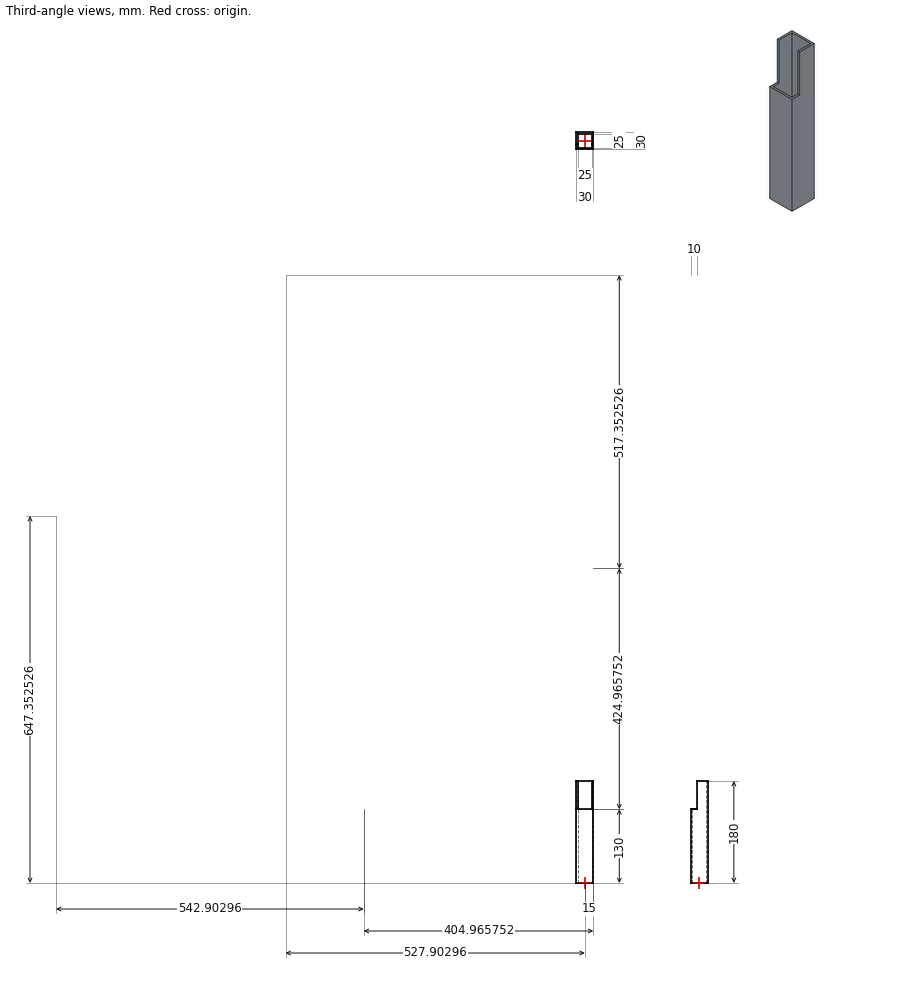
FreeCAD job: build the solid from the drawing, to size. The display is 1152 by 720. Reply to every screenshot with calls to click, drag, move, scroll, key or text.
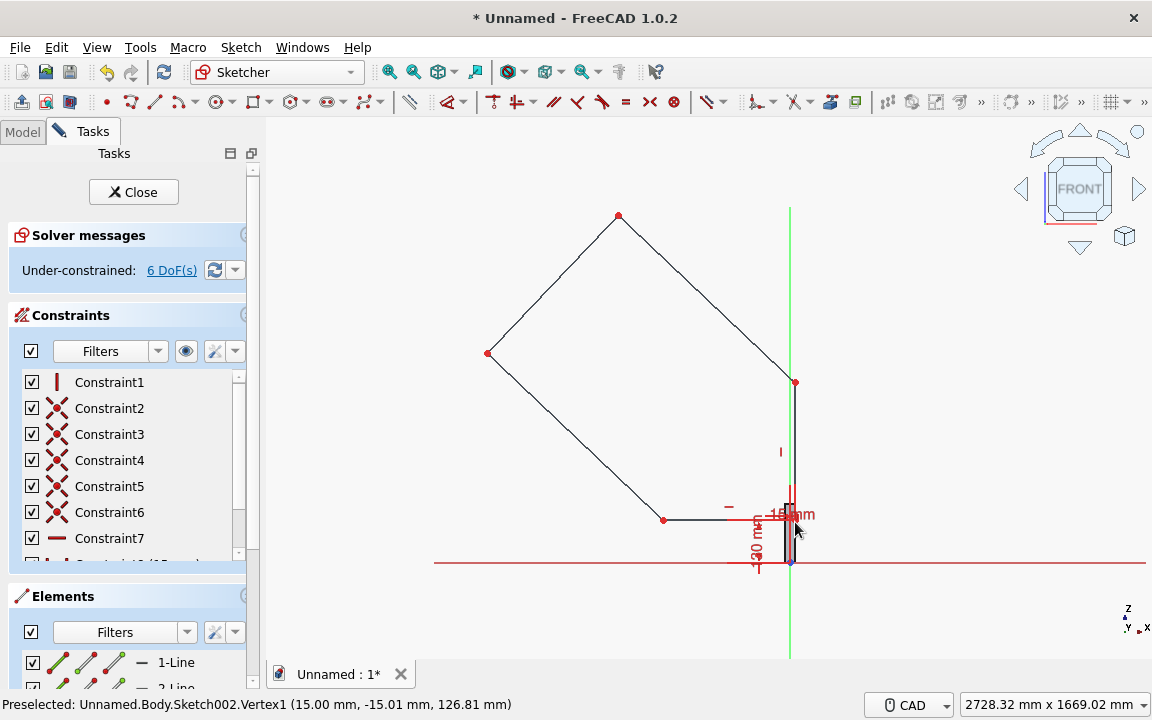
scroll(795, 479, up, 6)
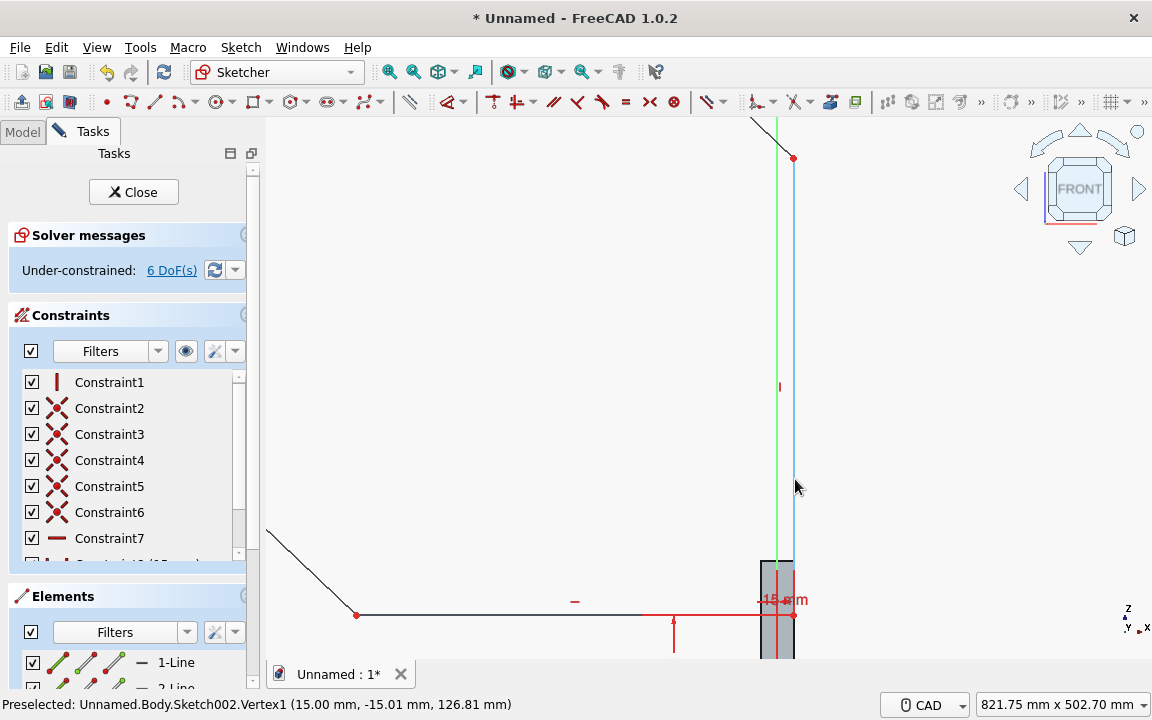
click(794, 478)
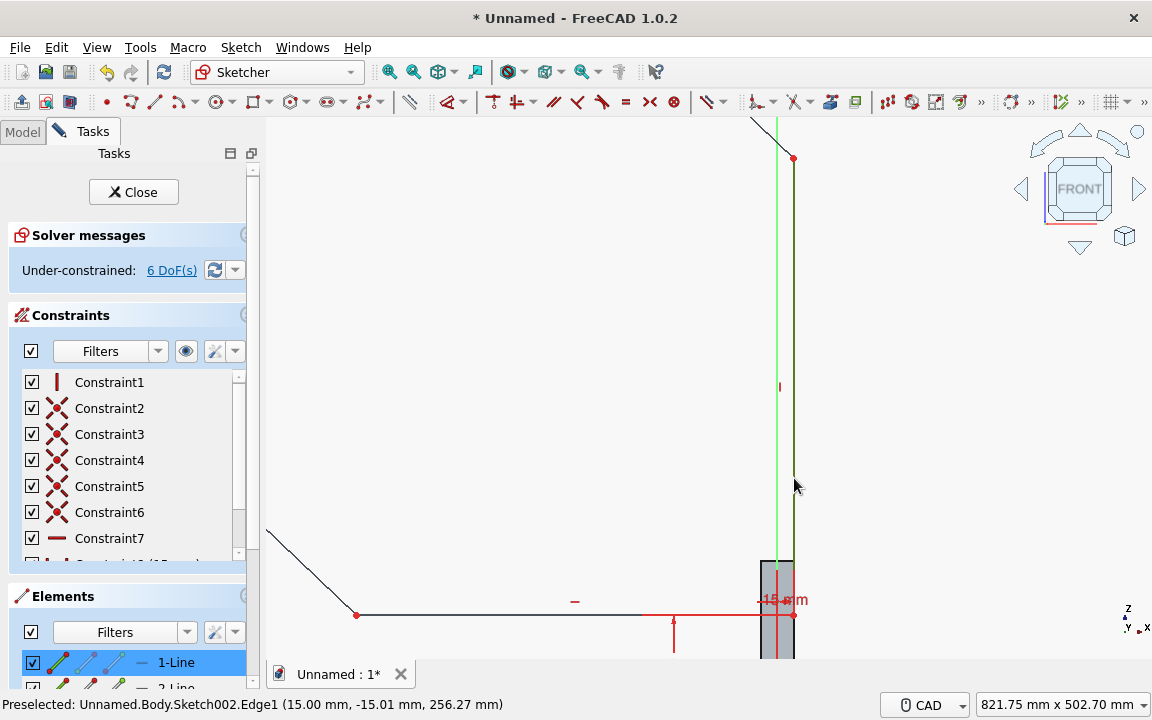
click(466, 102)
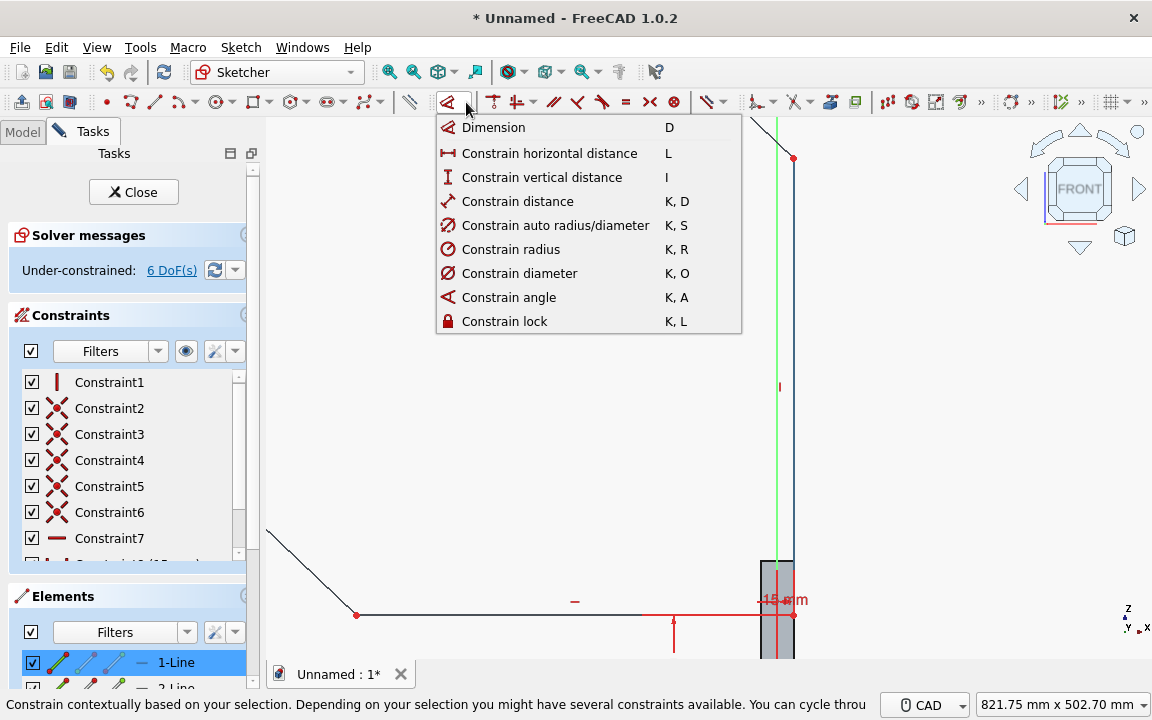
click(589, 177)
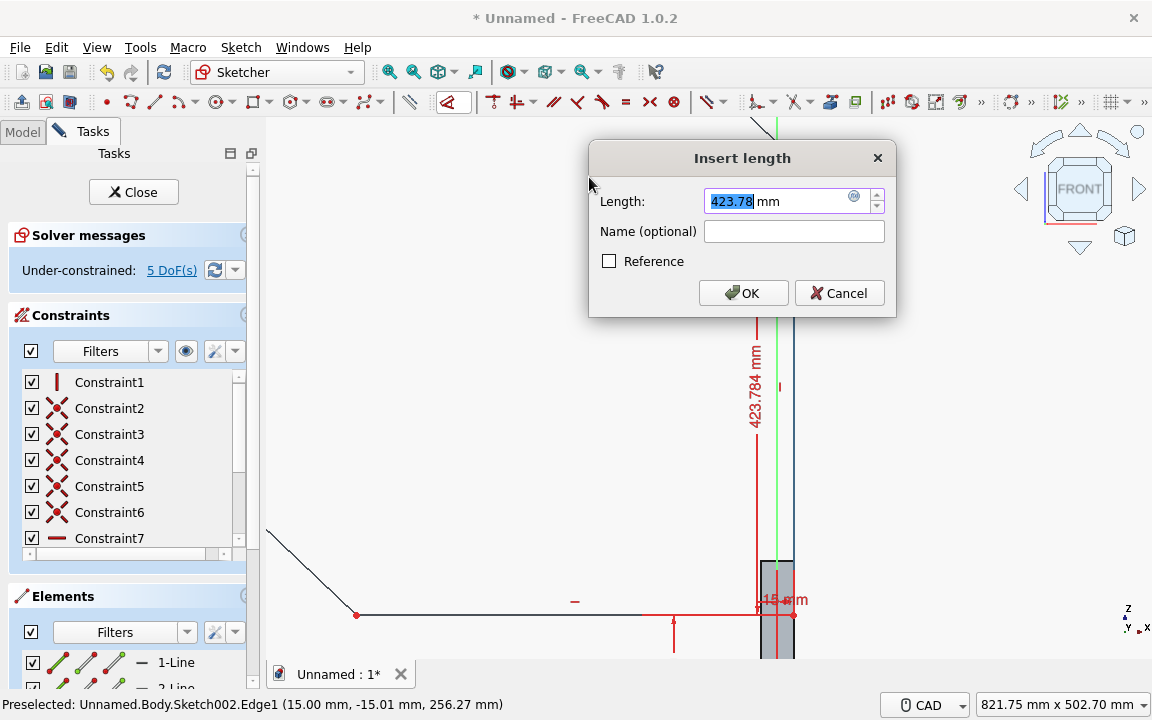
text(424.965752)
key(Return)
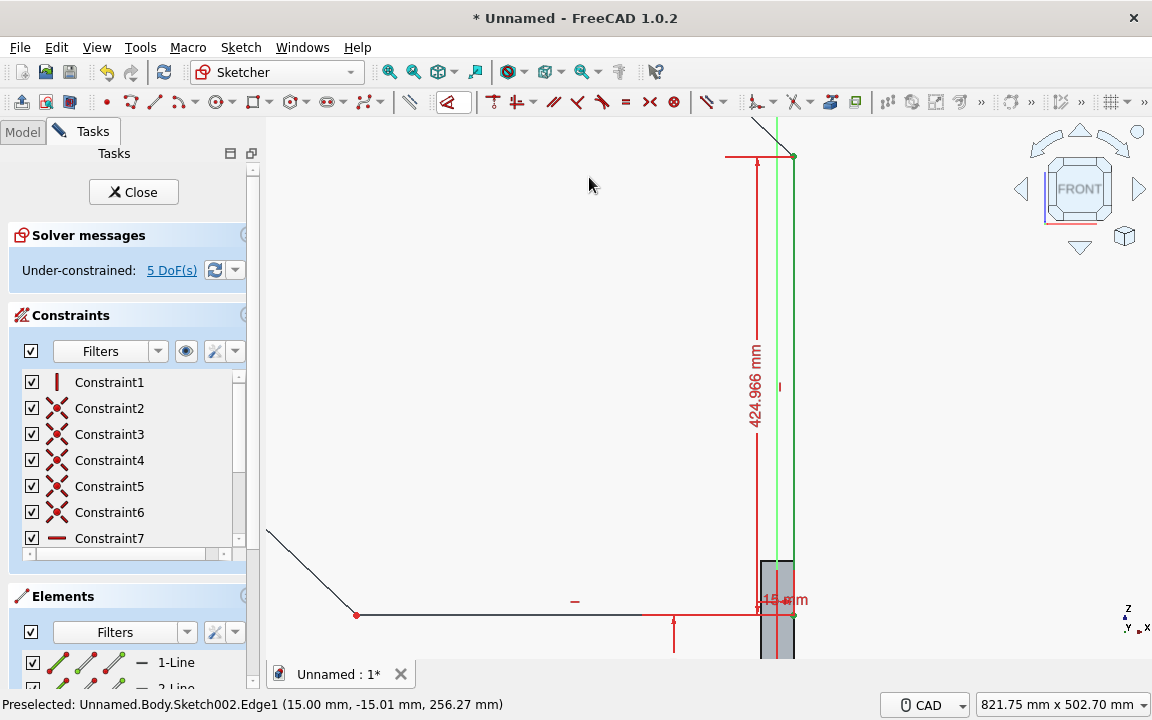
click(488, 615)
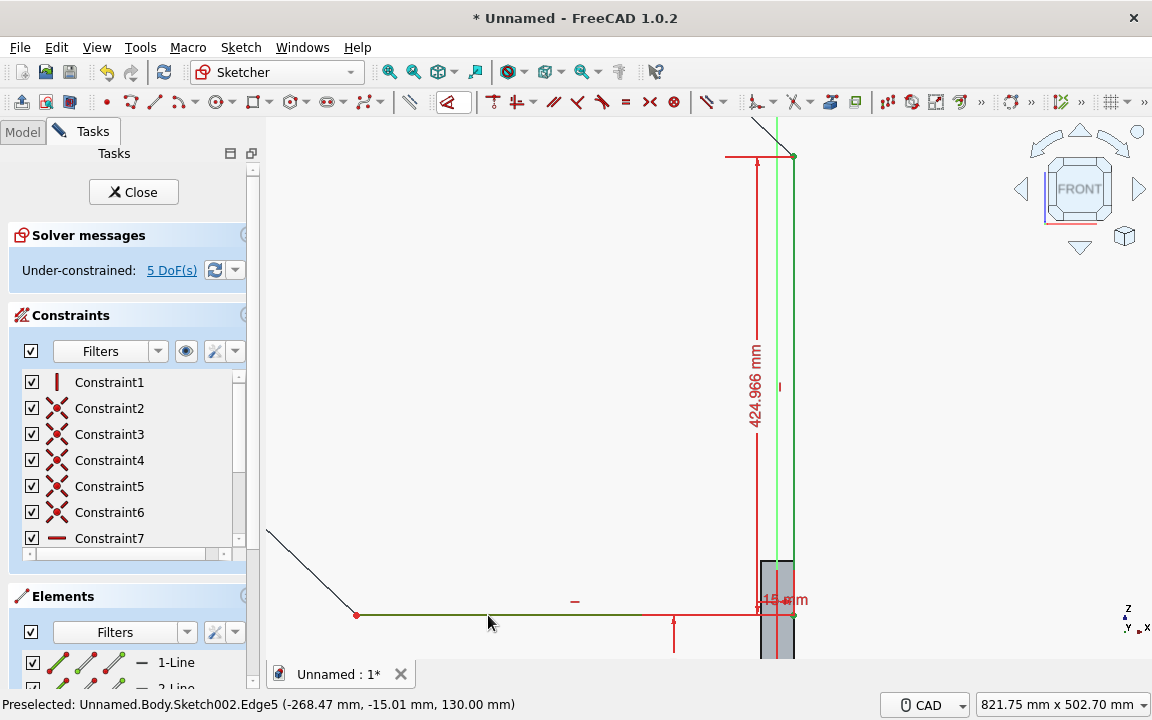
key(l)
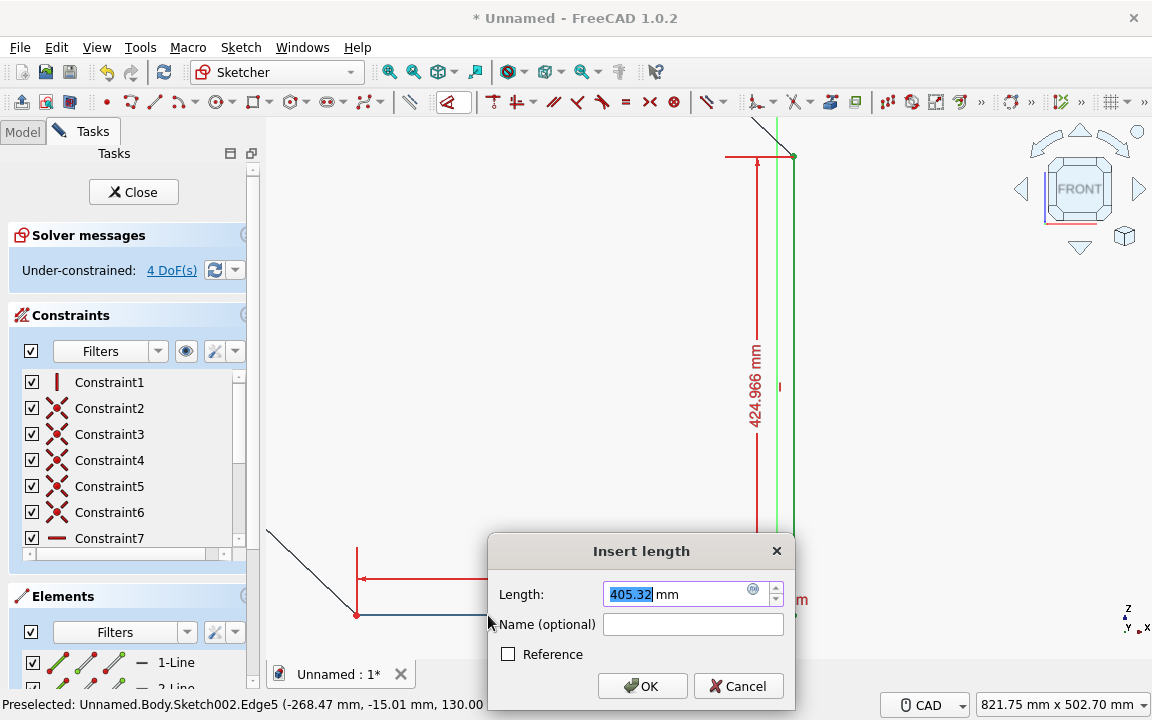
text(404.965752)
key(Return)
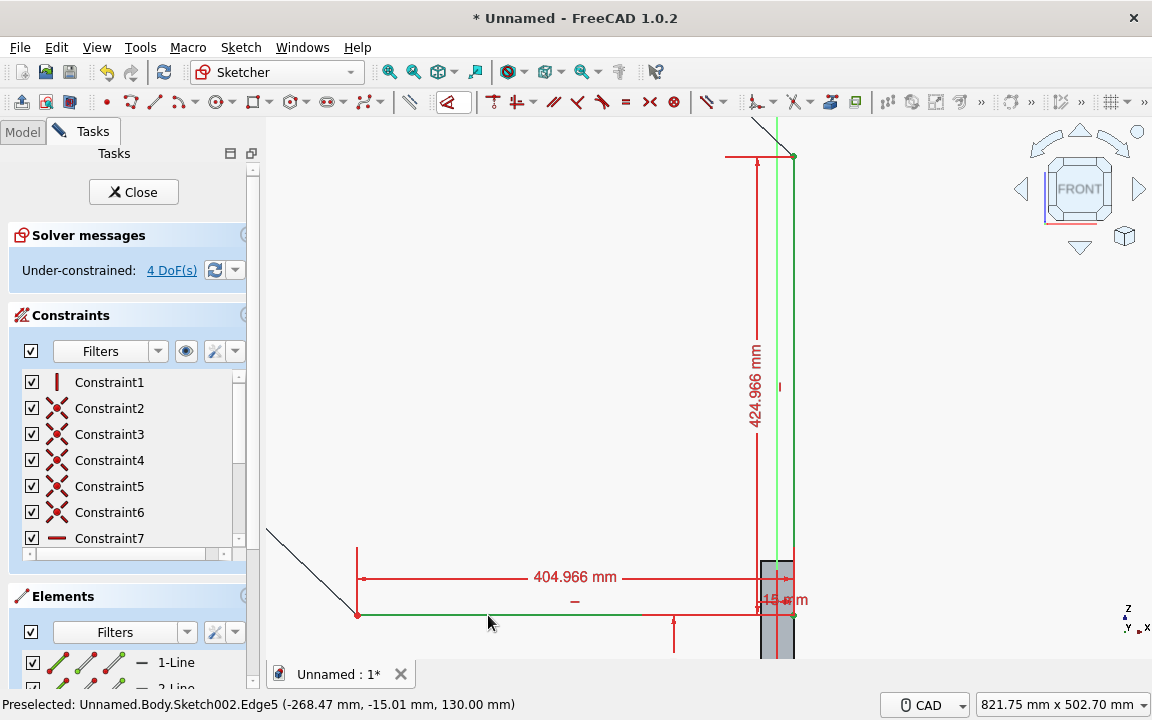
scroll(795, 479, down, 6)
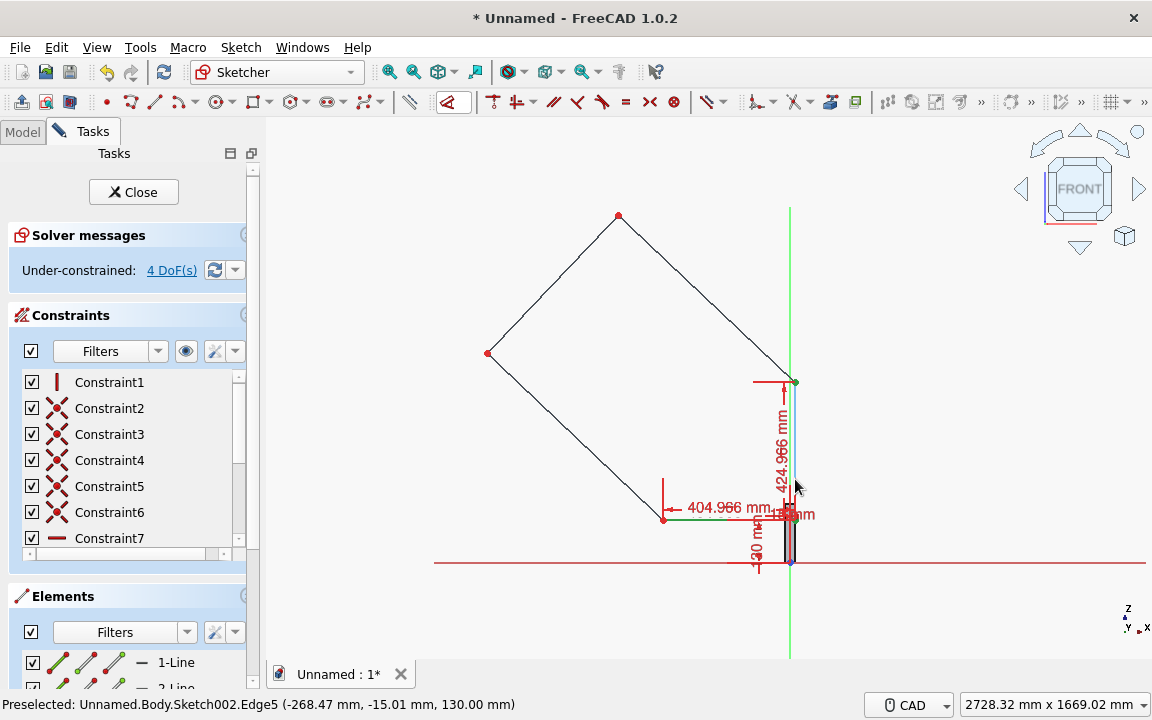
click(618, 216)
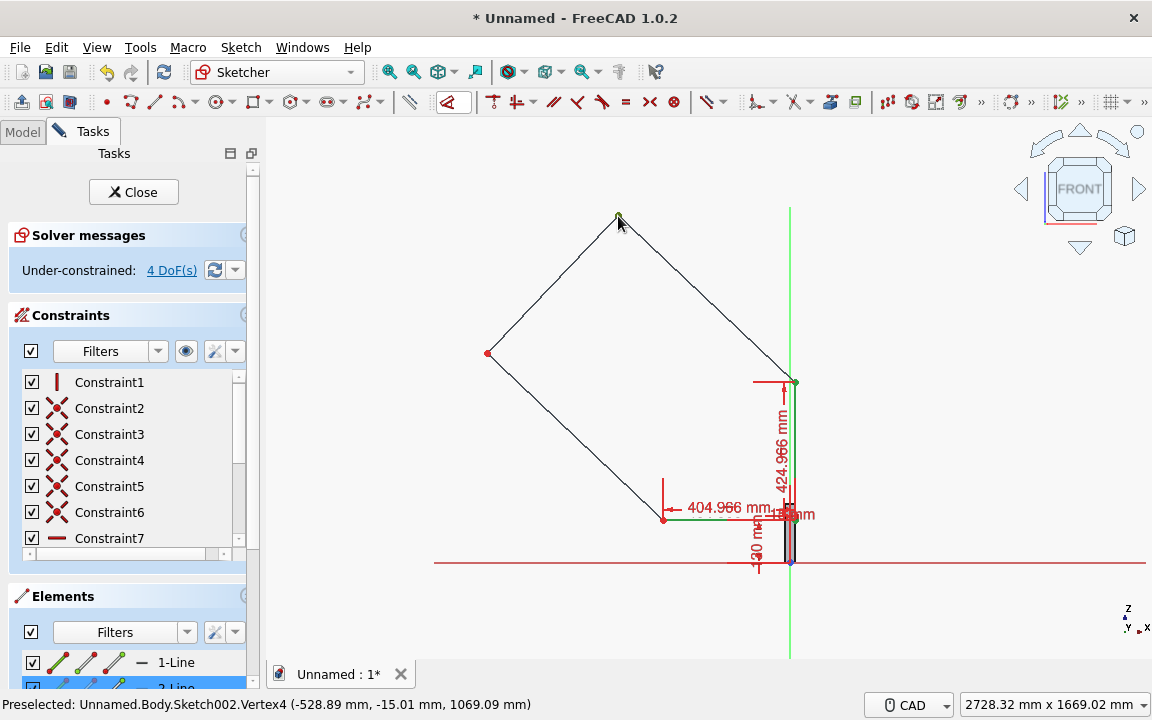
key(l)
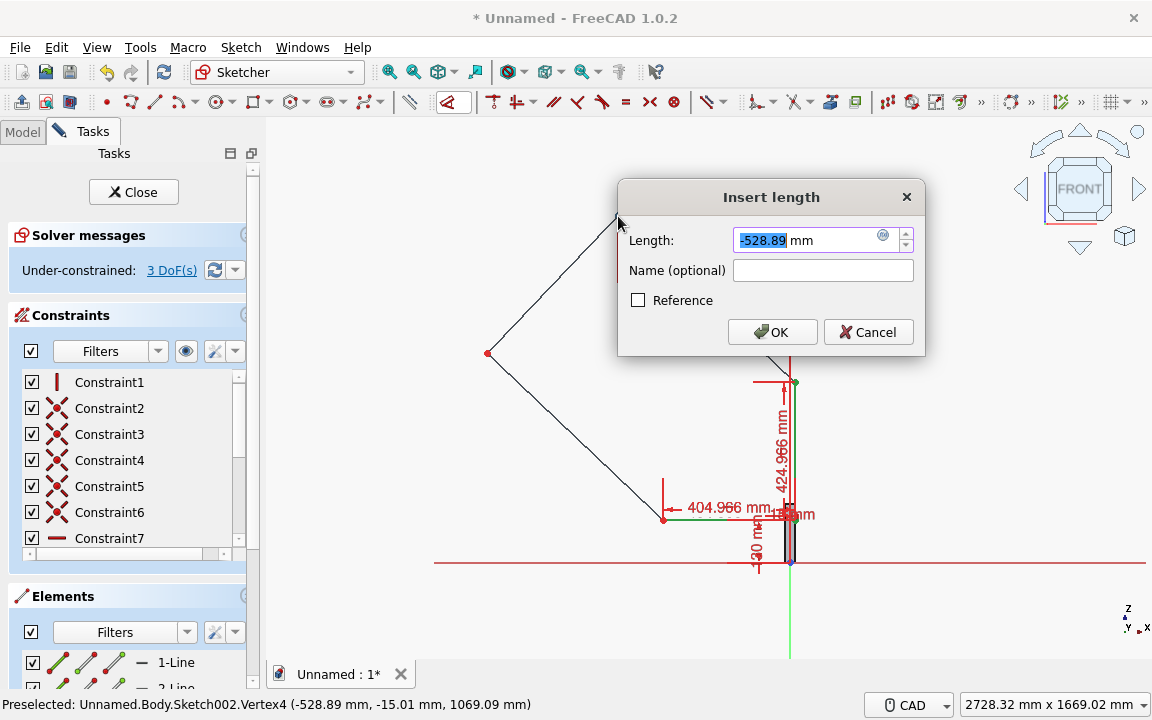
text(-527.90296)
key(Return)